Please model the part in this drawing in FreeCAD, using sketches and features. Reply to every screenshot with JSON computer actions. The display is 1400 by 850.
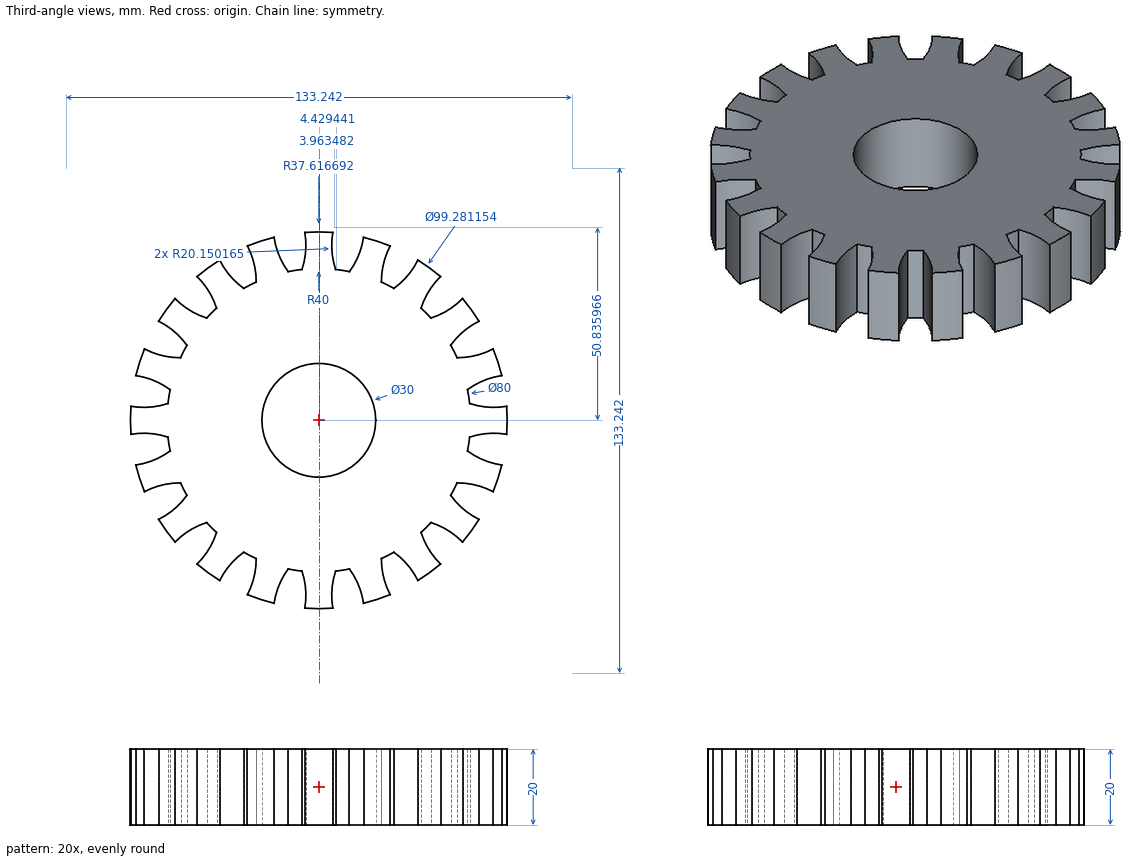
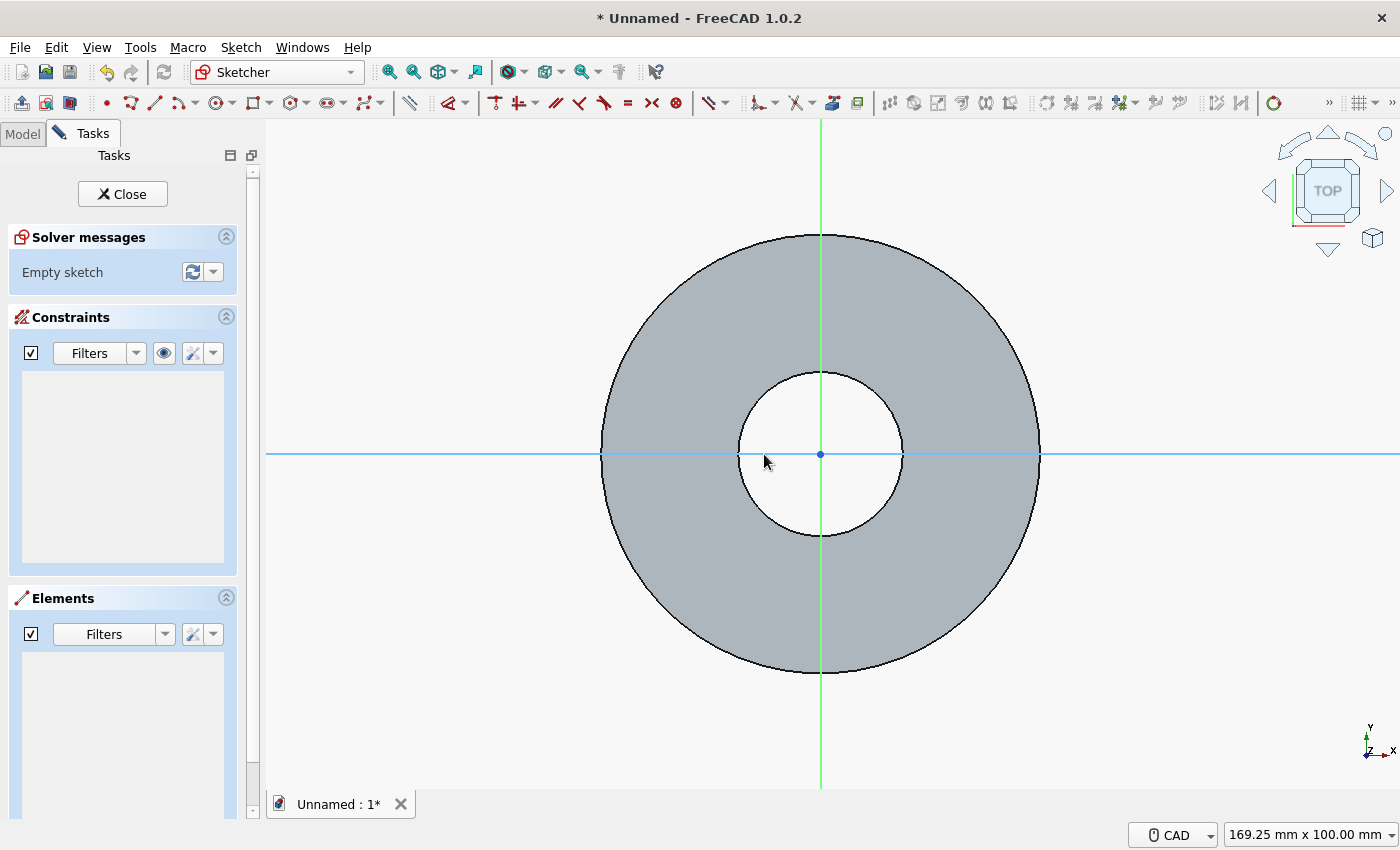
{"action": "scroll", "coordinate": [791, 335], "scroll_direction": "up", "scroll_amount": 14}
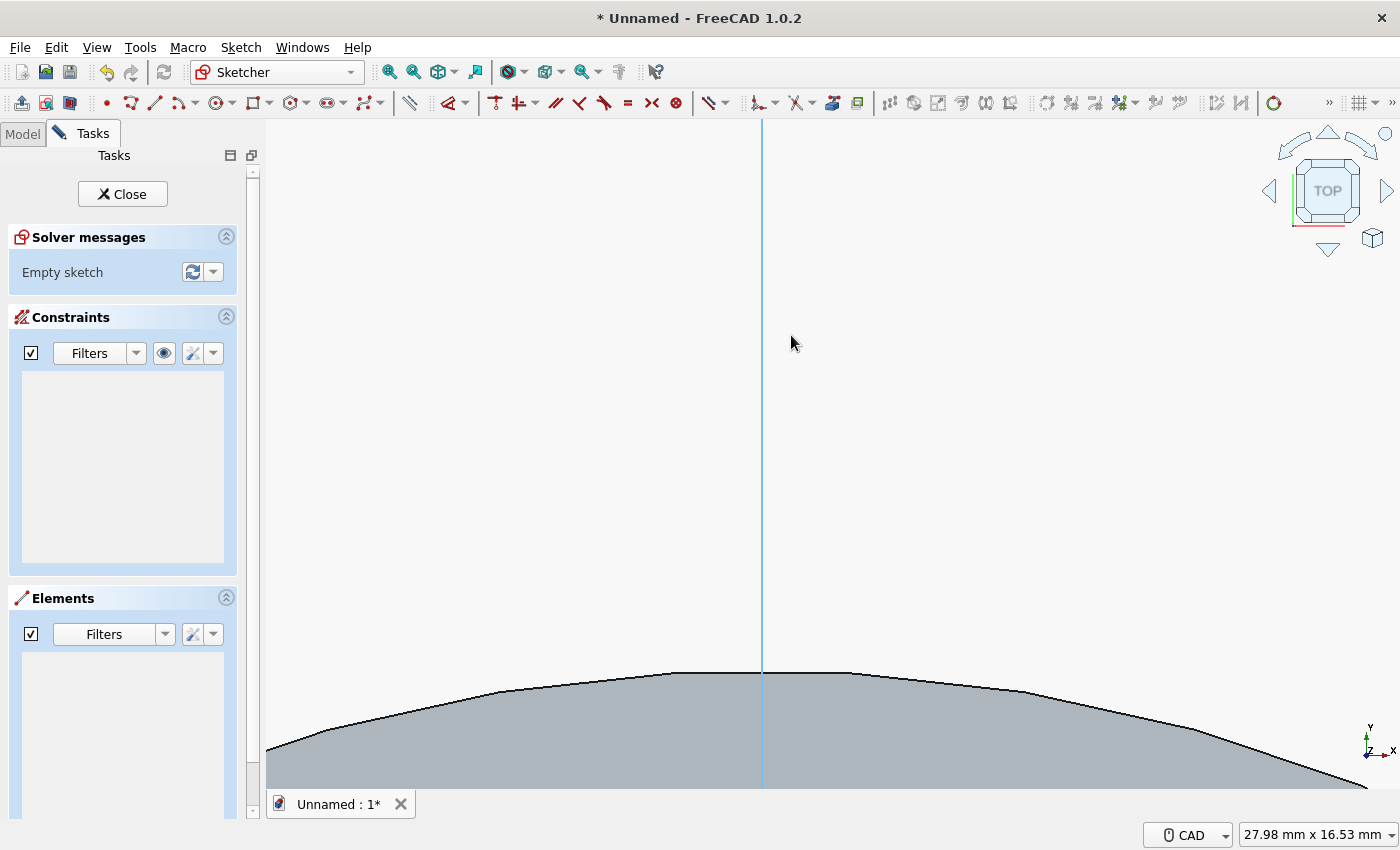
{"action": "key", "text": "g 3 a"}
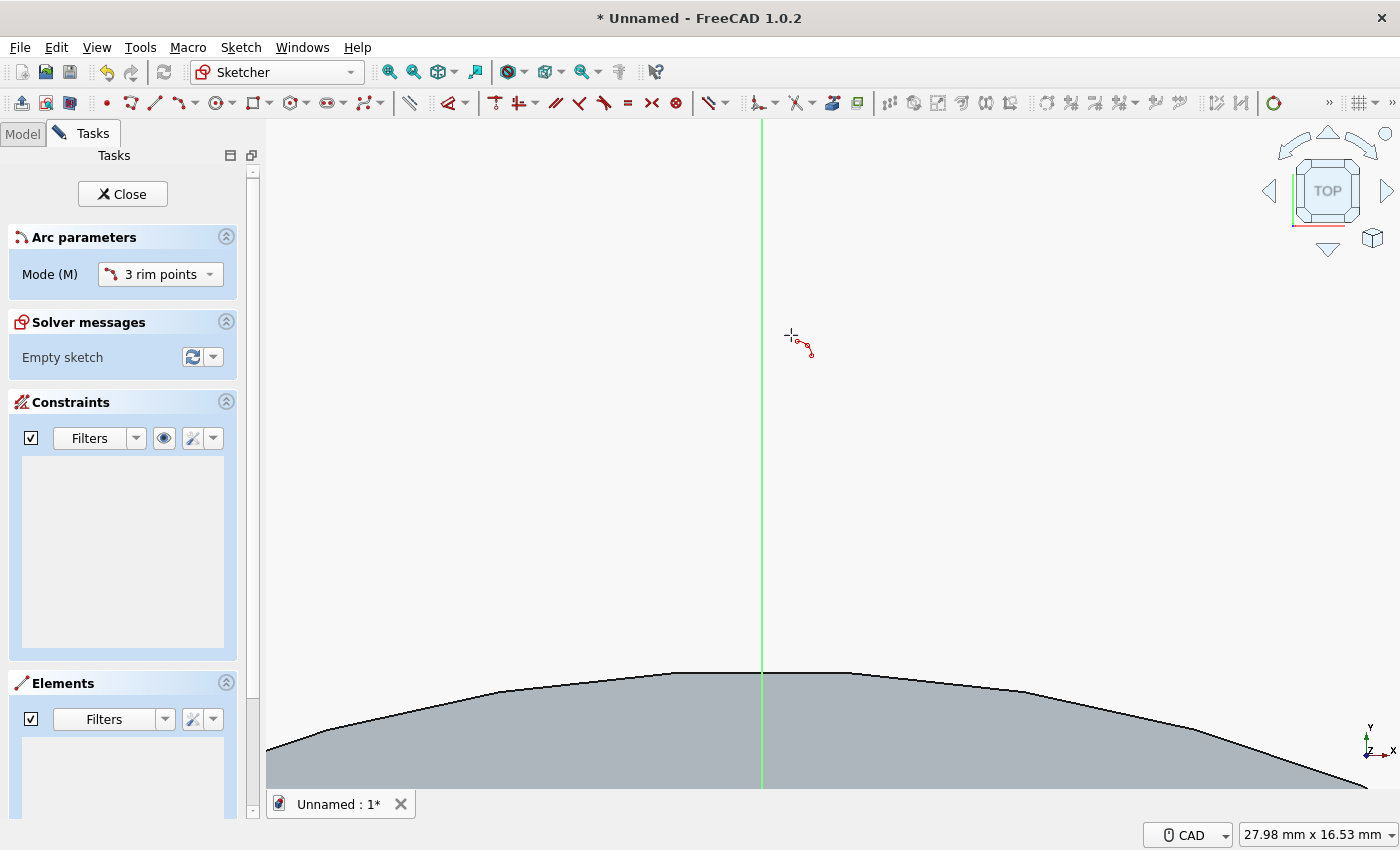
{"action": "left_click", "coordinate": [941, 681]}
{"action": "left_click", "coordinate": [922, 232]}
{"action": "left_click", "coordinate": [900, 458]}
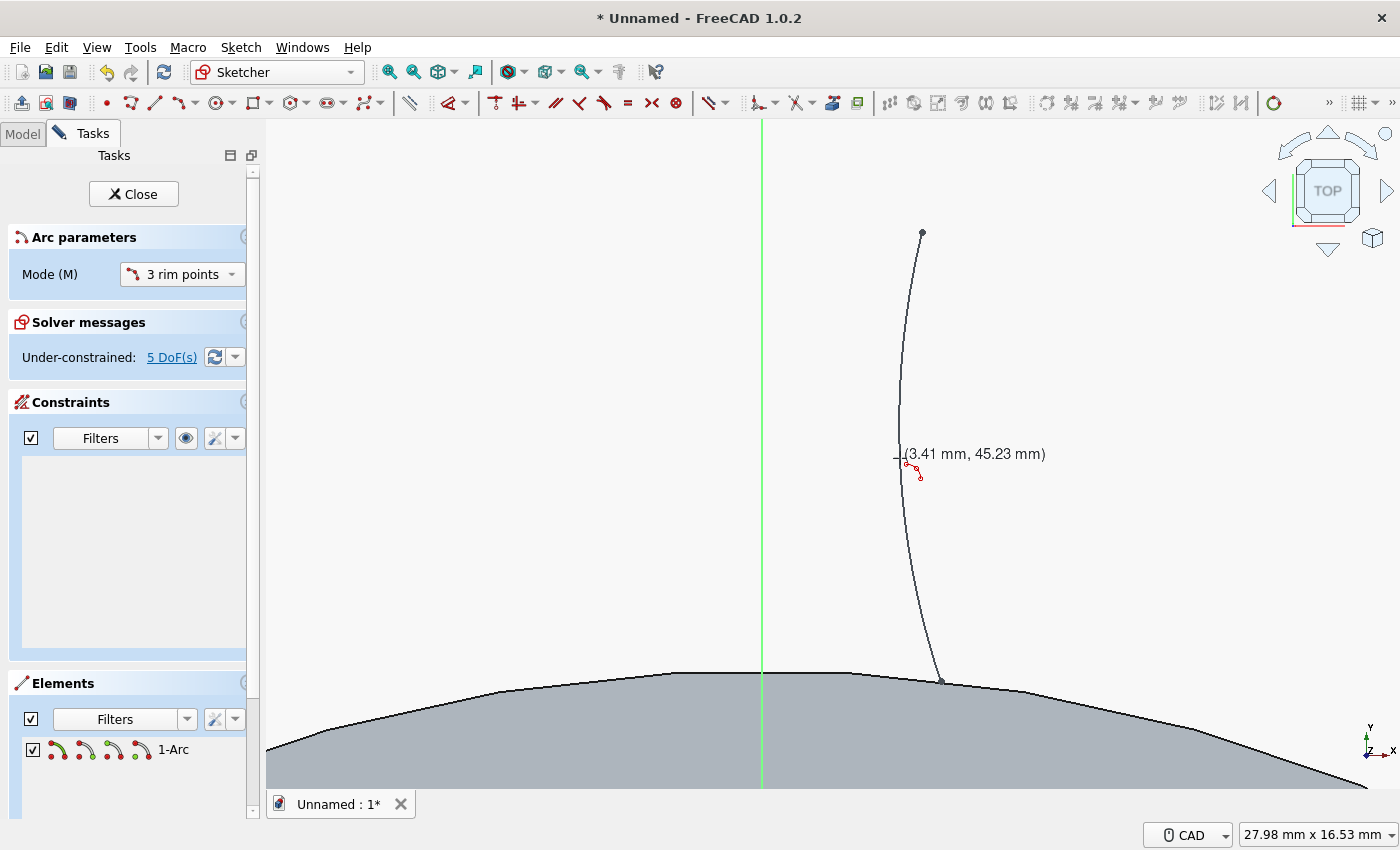
{"action": "left_click", "coordinate": [922, 233]}
{"action": "left_click", "coordinate": [601, 232]}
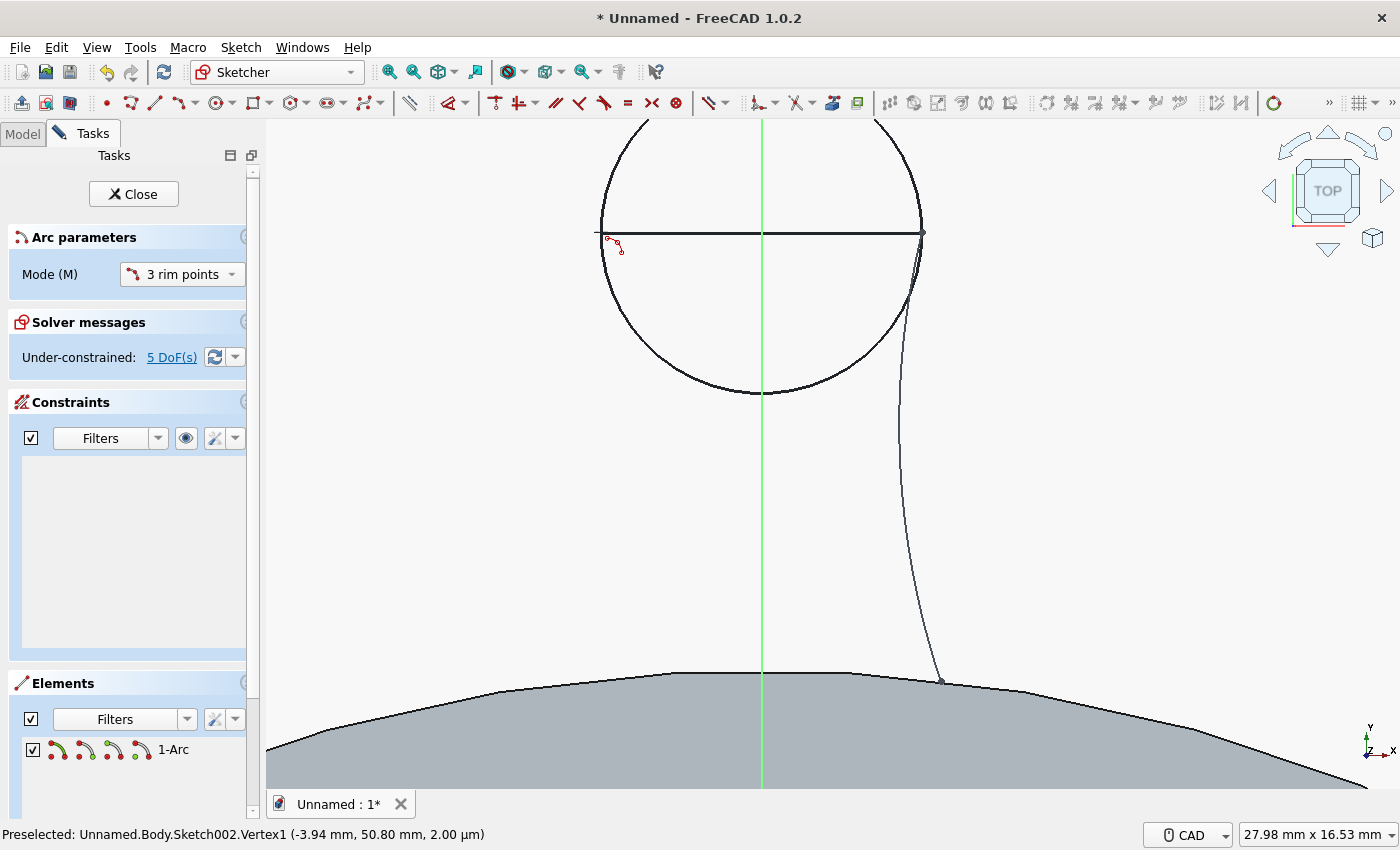
{"action": "scroll", "coordinate": [794, 223], "scroll_direction": "up", "scroll_amount": 4}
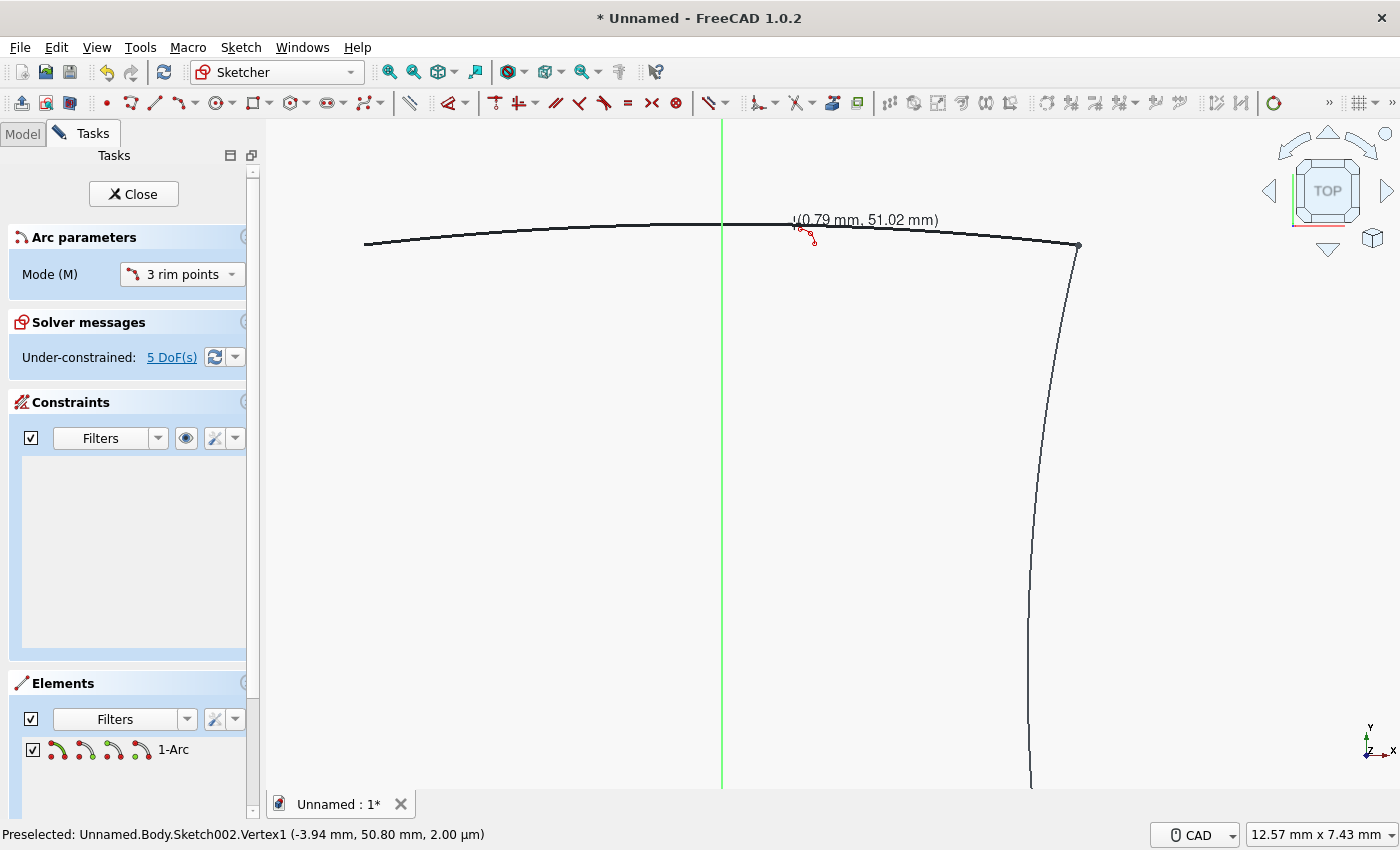
{"action": "left_click", "coordinate": [793, 224]}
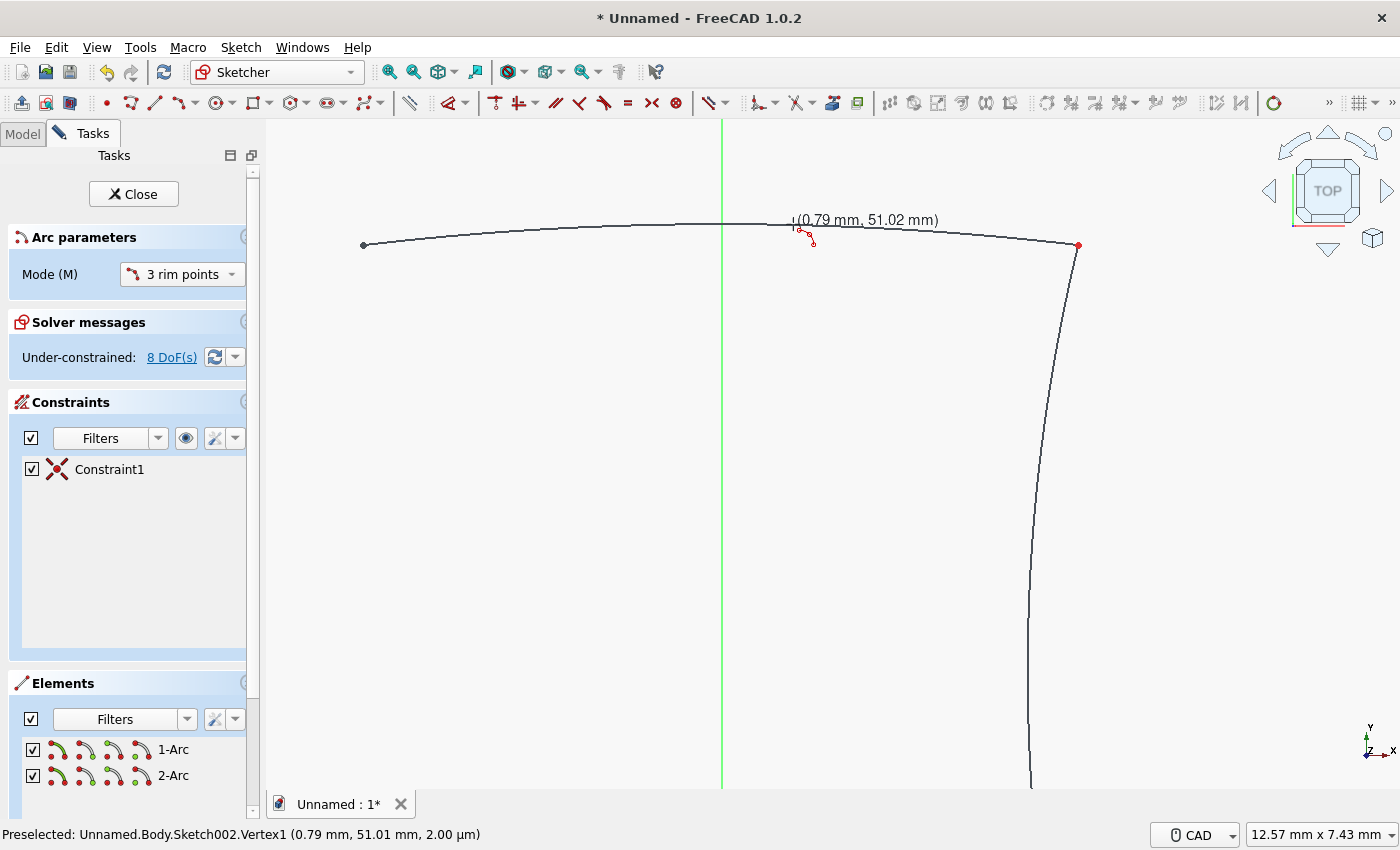
{"action": "left_click", "coordinate": [364, 245]}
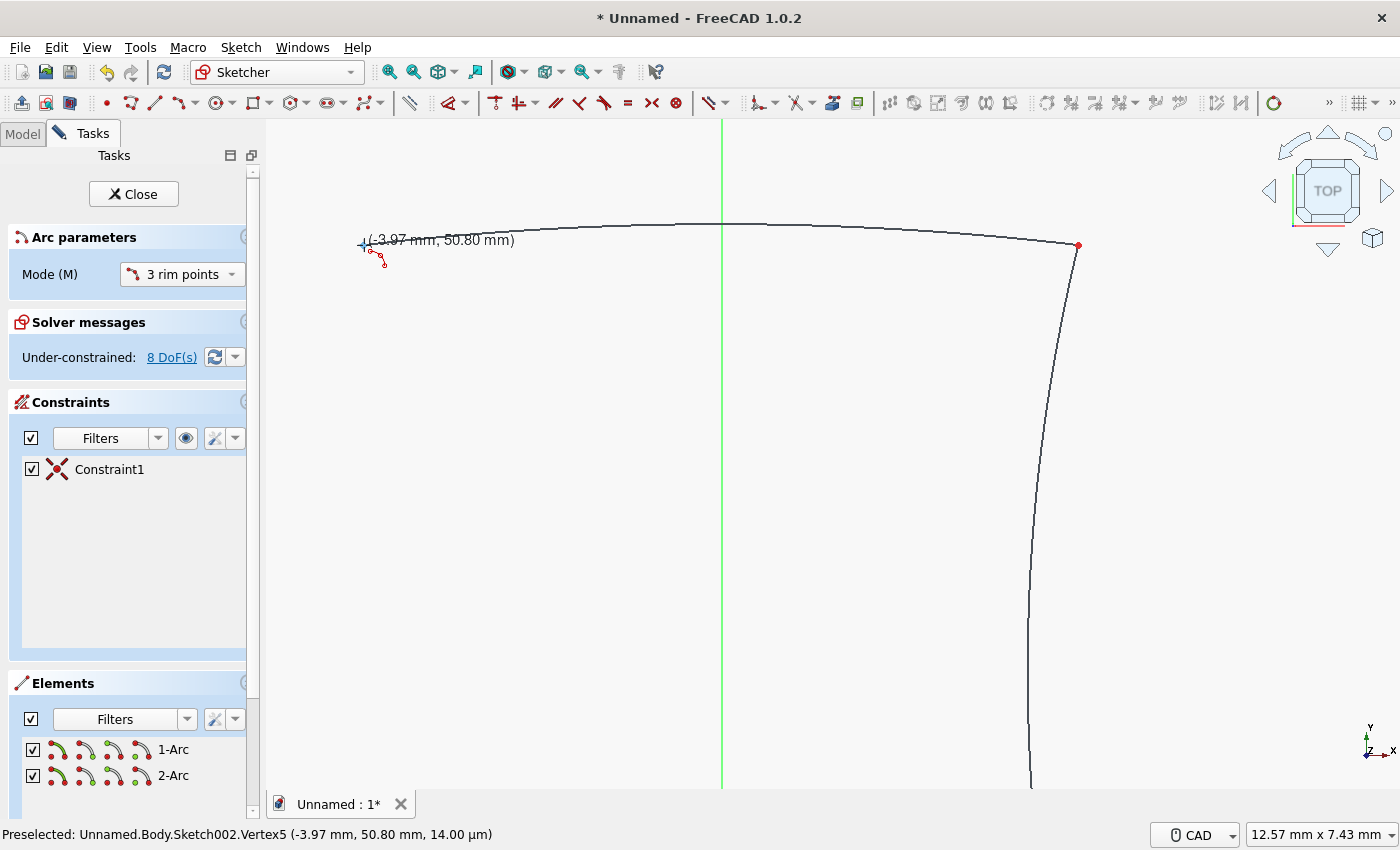
{"action": "scroll", "coordinate": [799, 227], "scroll_direction": "down", "scroll_amount": 4}